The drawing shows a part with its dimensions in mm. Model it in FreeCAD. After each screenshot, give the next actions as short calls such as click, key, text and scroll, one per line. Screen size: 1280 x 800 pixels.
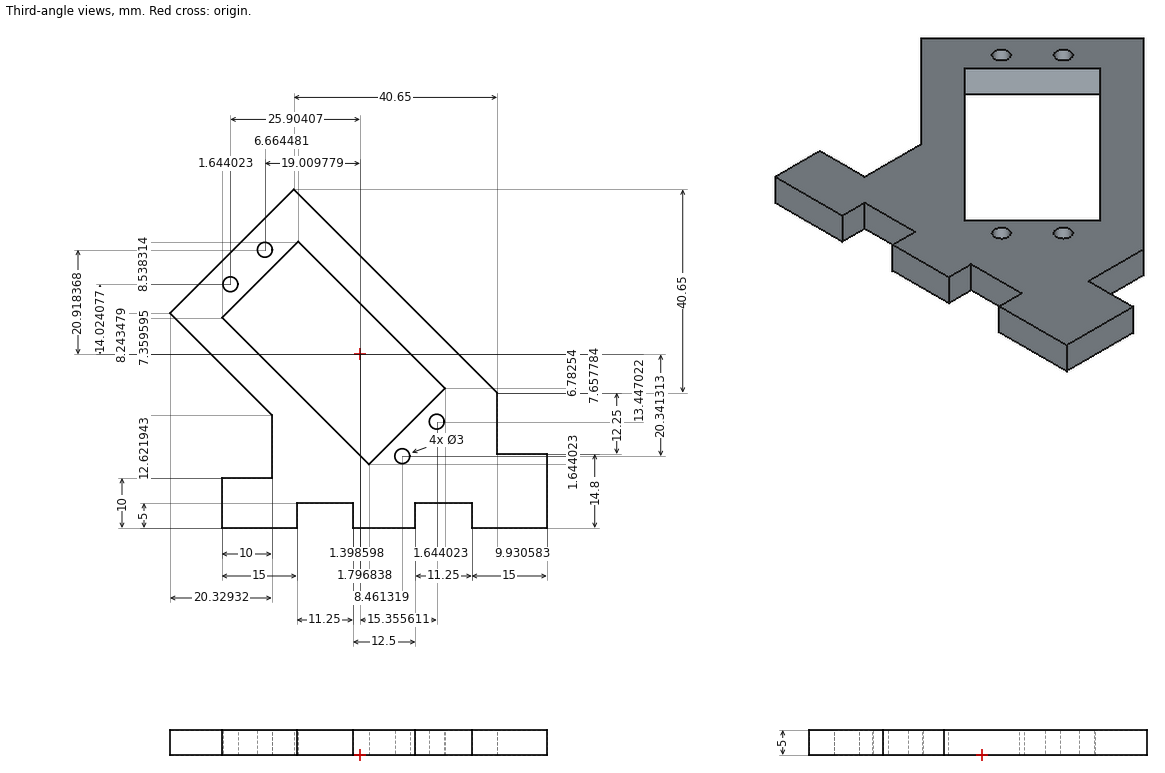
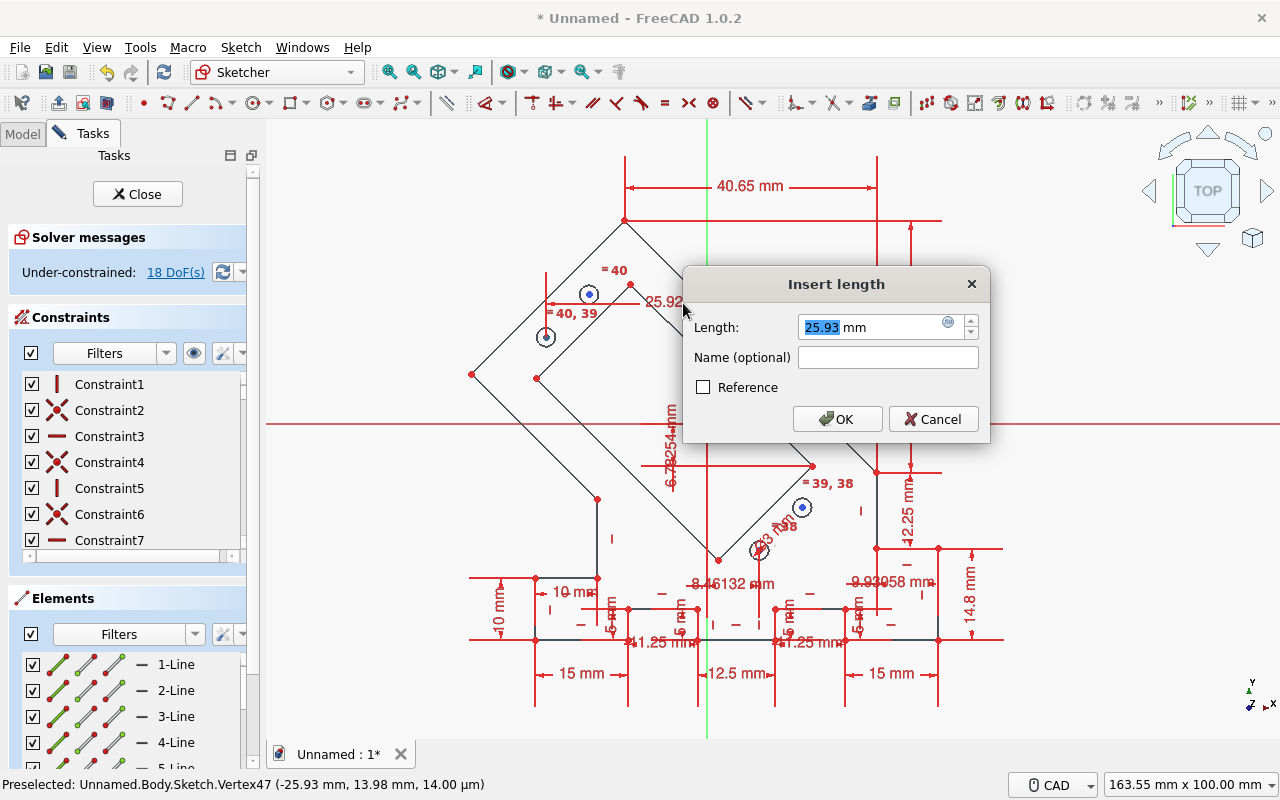
text(25.90407)
key(Return)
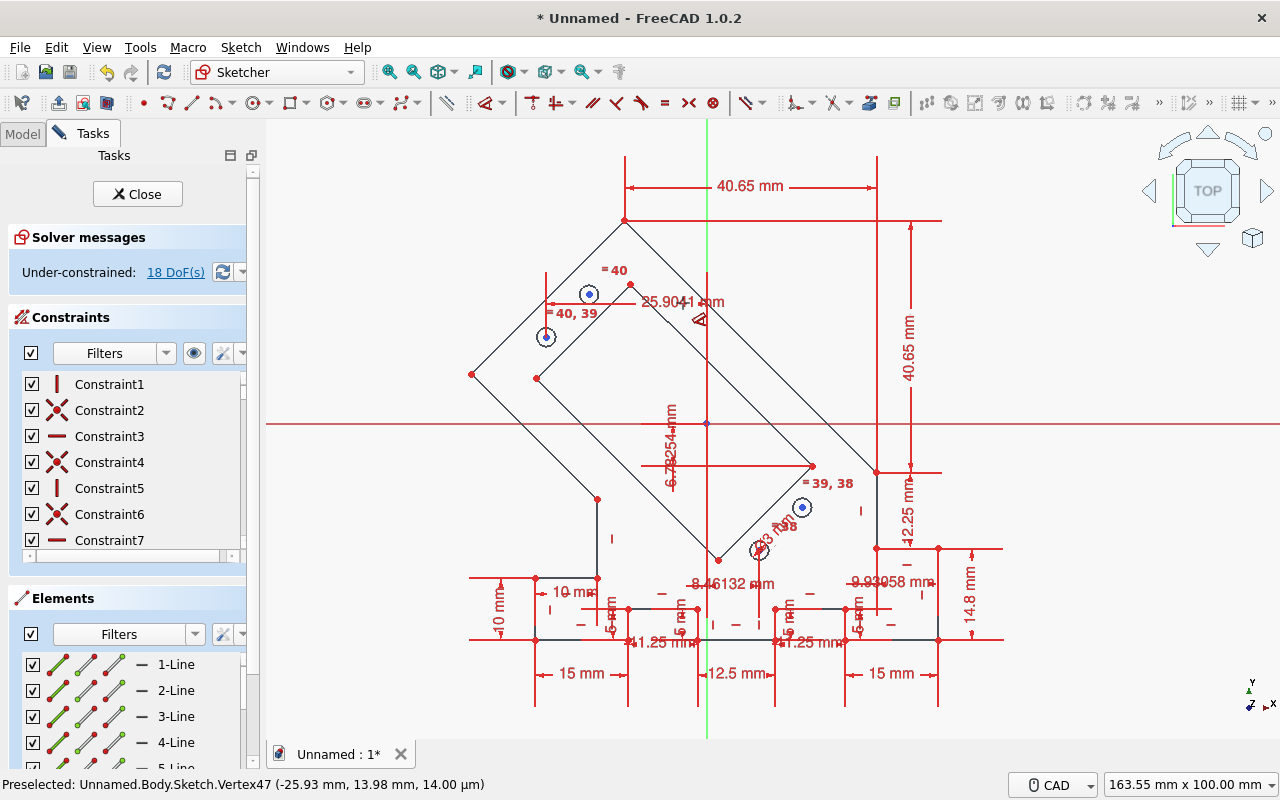
click(597, 523)
click(563, 539)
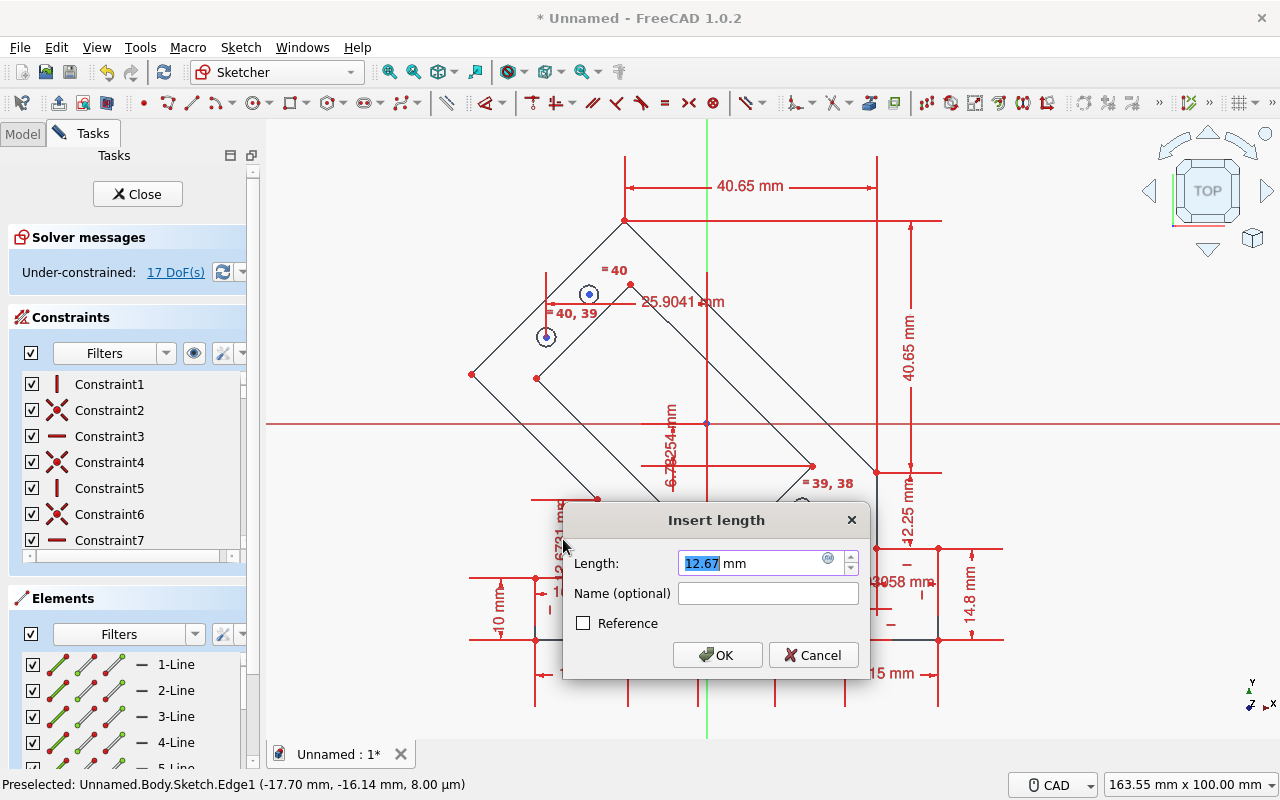
text(12.621943)
key(Return)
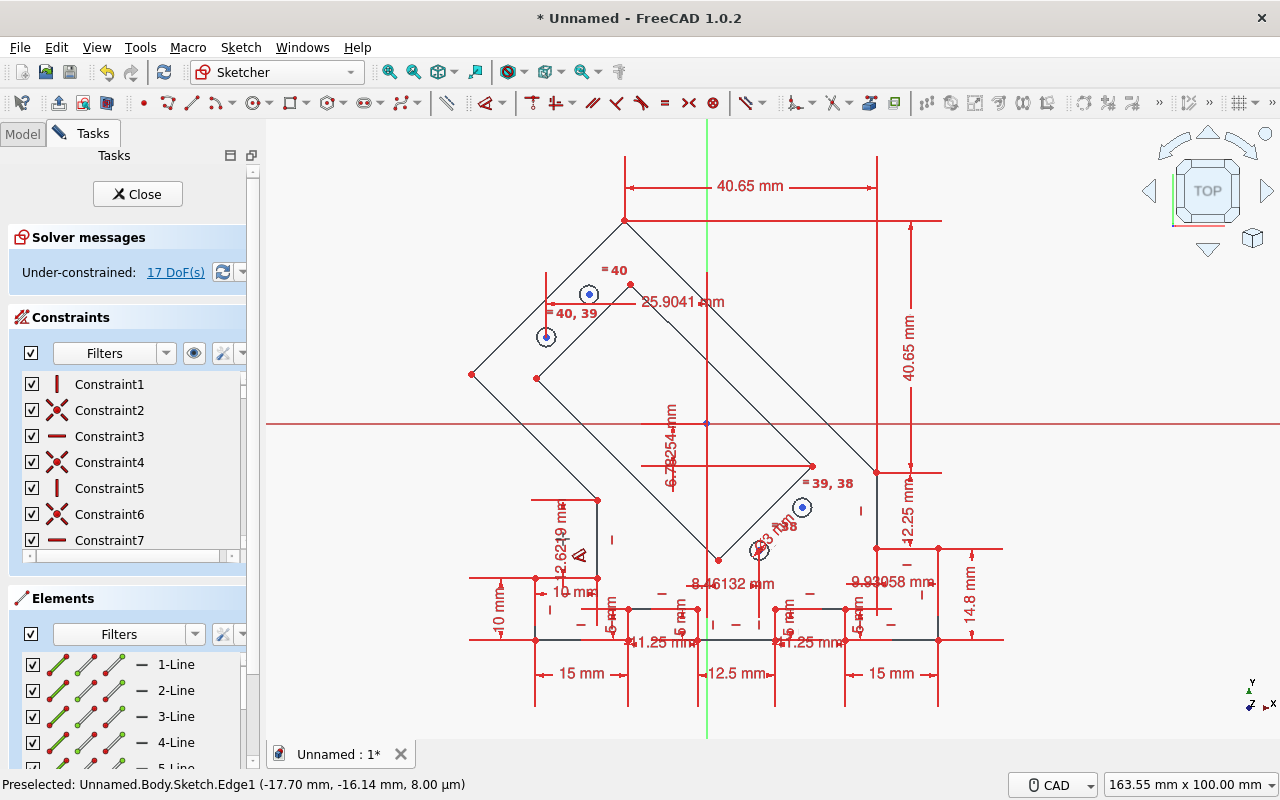
scroll(698, 609, up, 8)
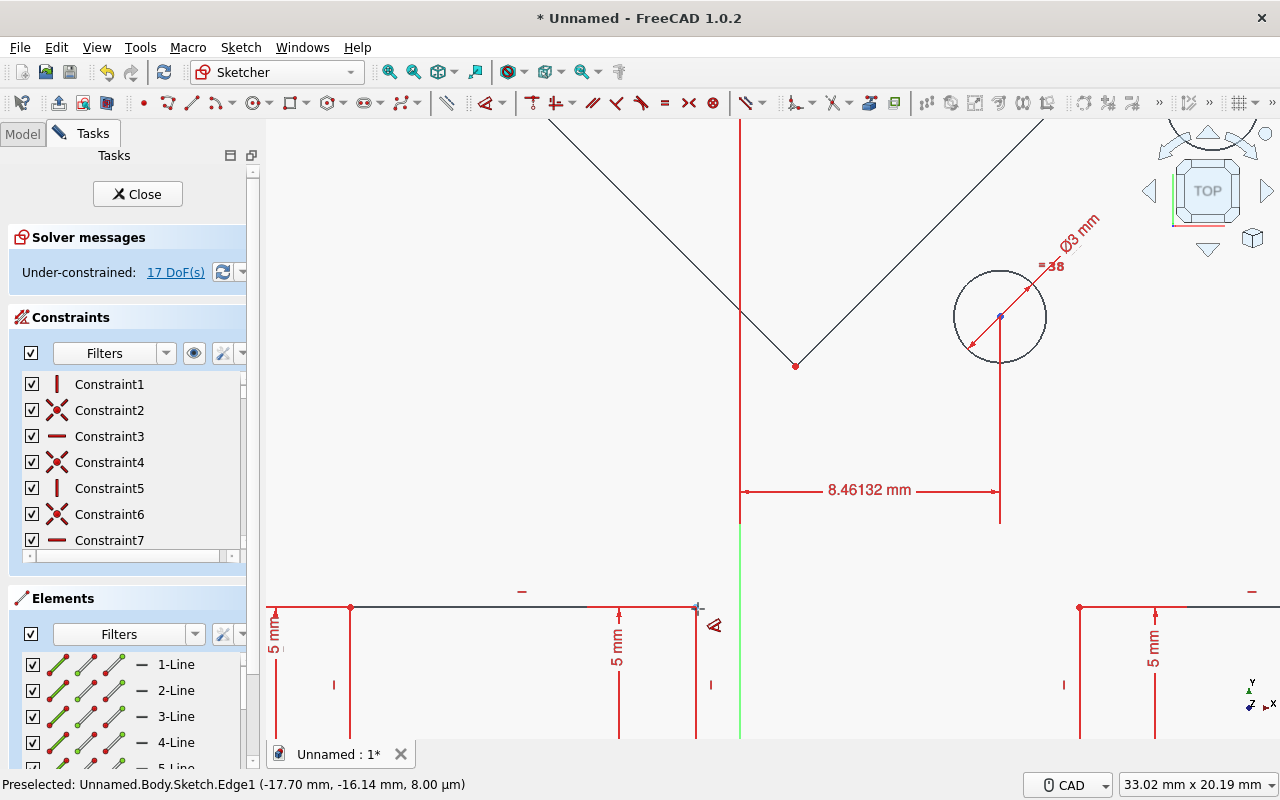
click(696, 607)
click(718, 641)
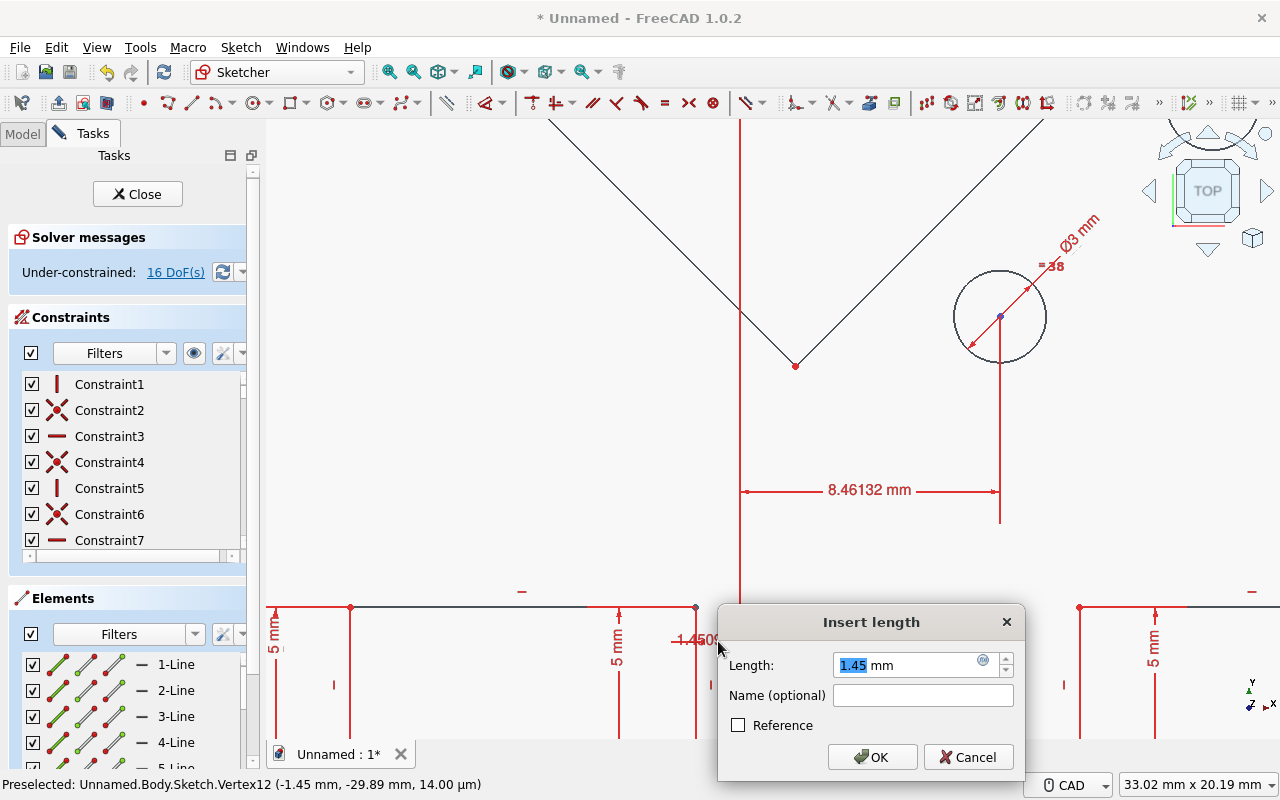
text(1.398598)
key(Return)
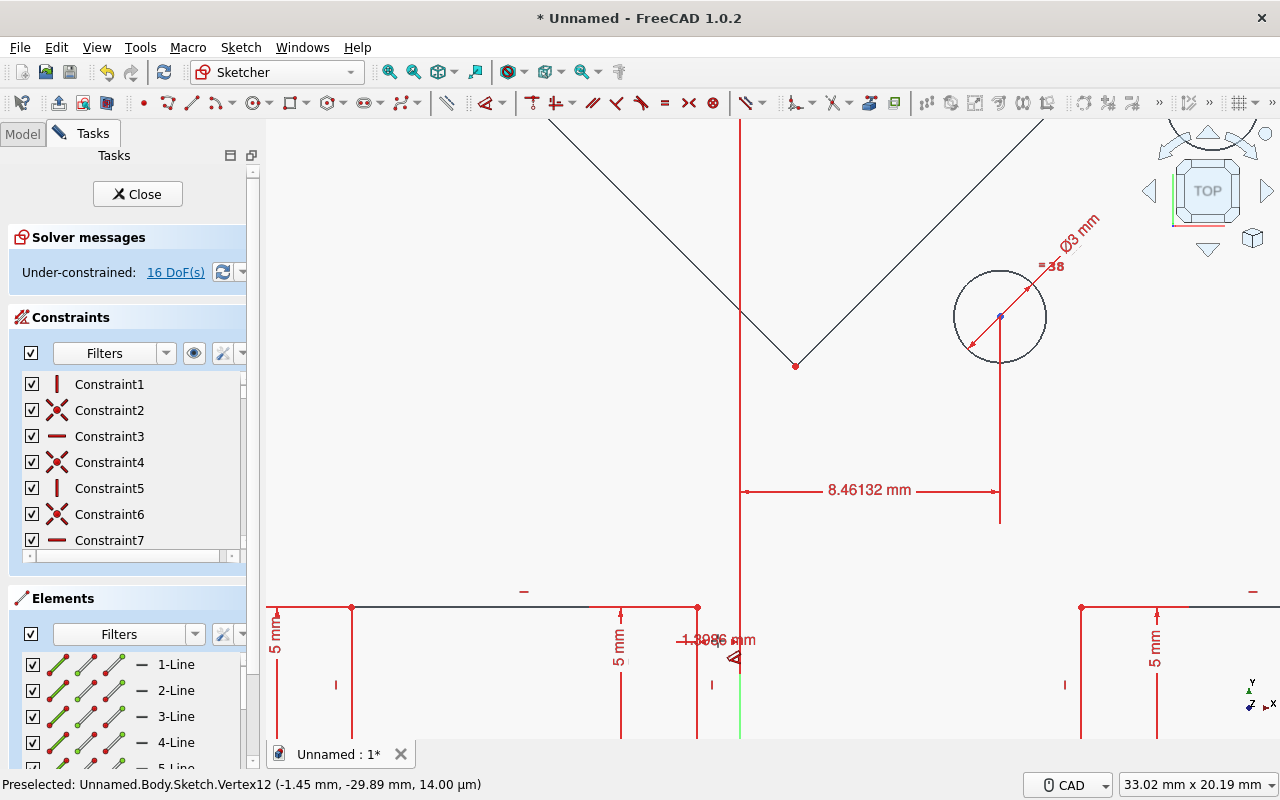
scroll(698, 609, down, 8)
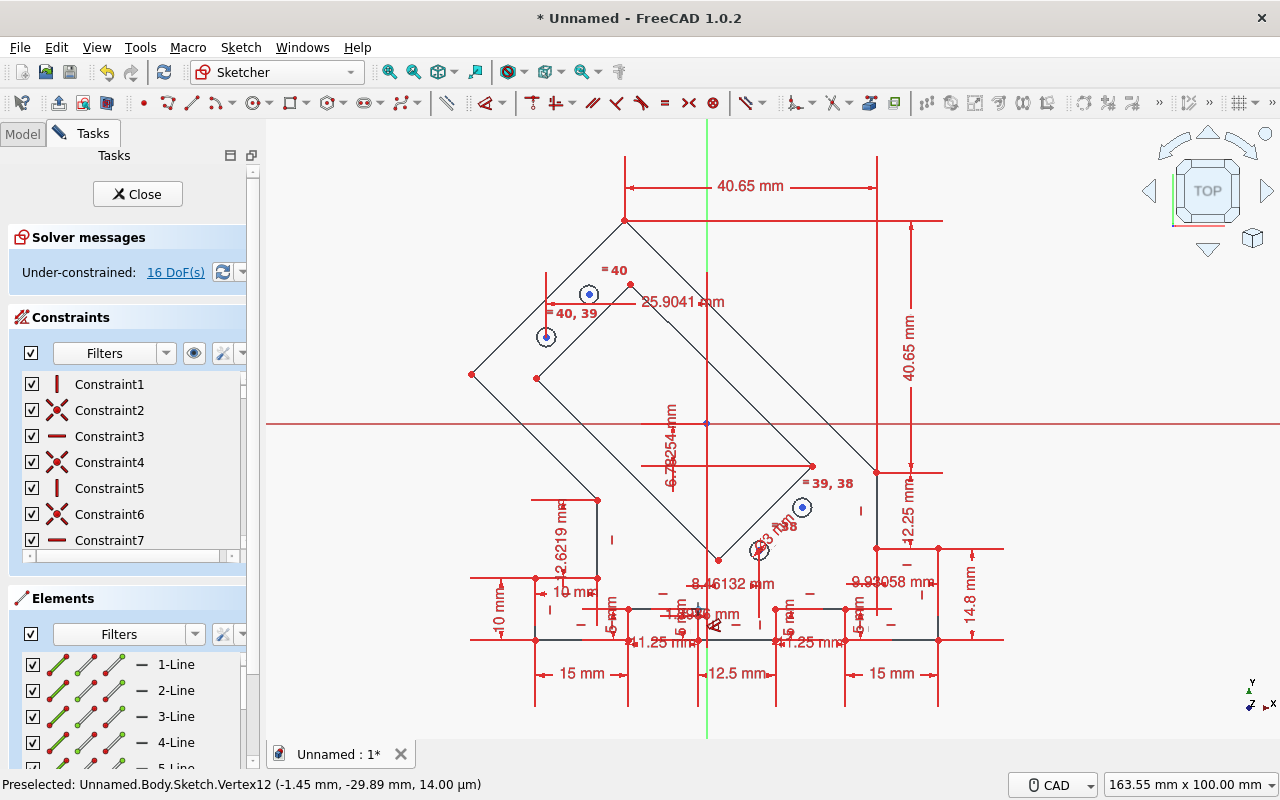
click(877, 473)
click(911, 448)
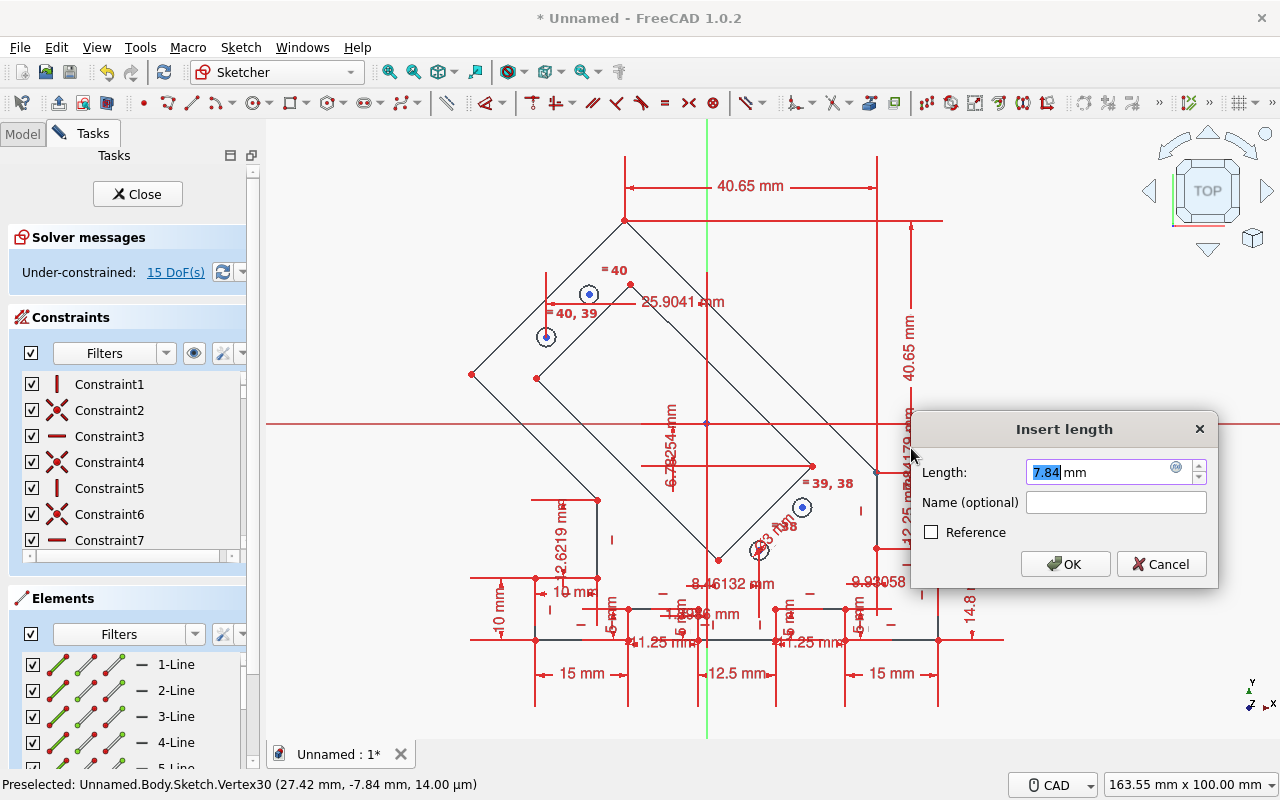
text(7.657784)
key(Return)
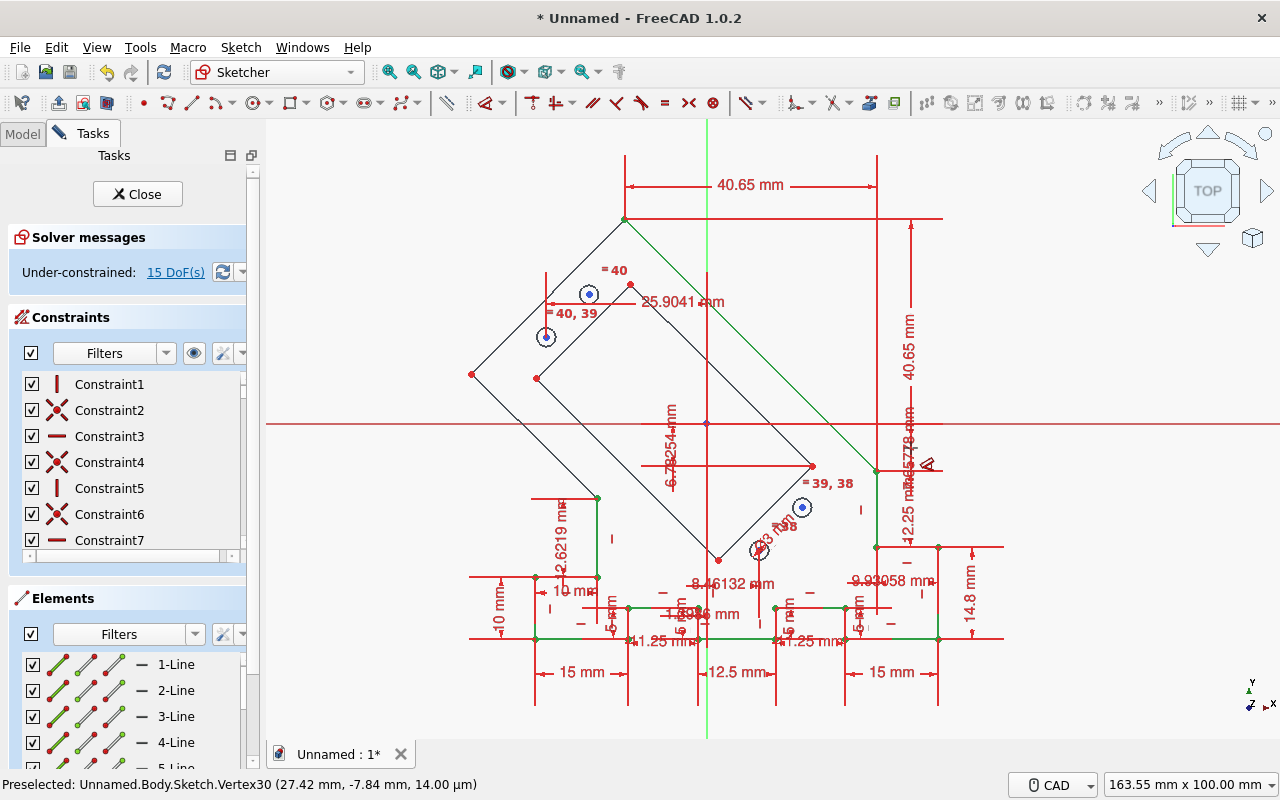
click(472, 374)
click(438, 399)